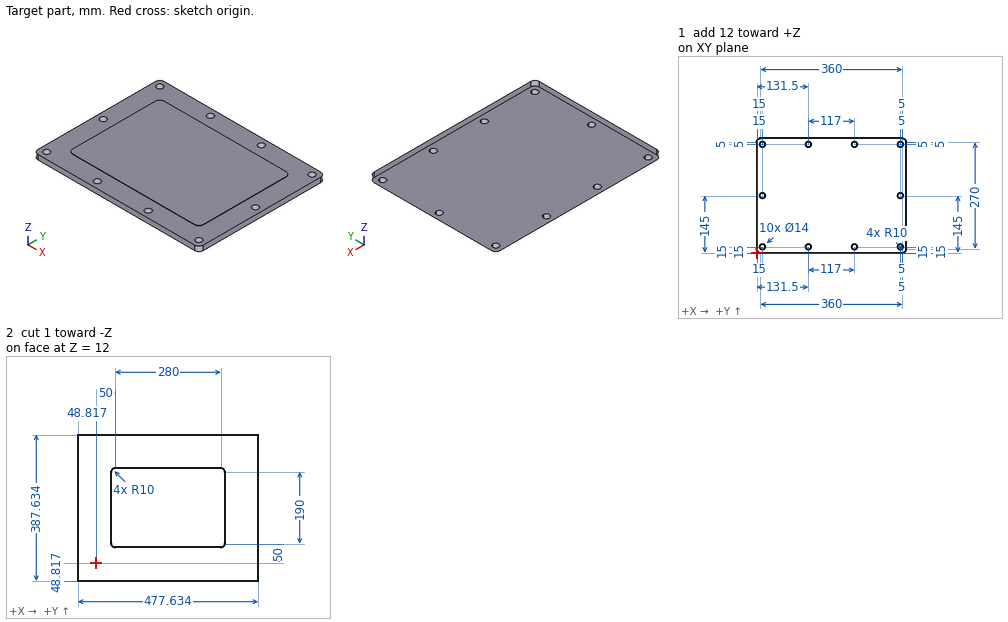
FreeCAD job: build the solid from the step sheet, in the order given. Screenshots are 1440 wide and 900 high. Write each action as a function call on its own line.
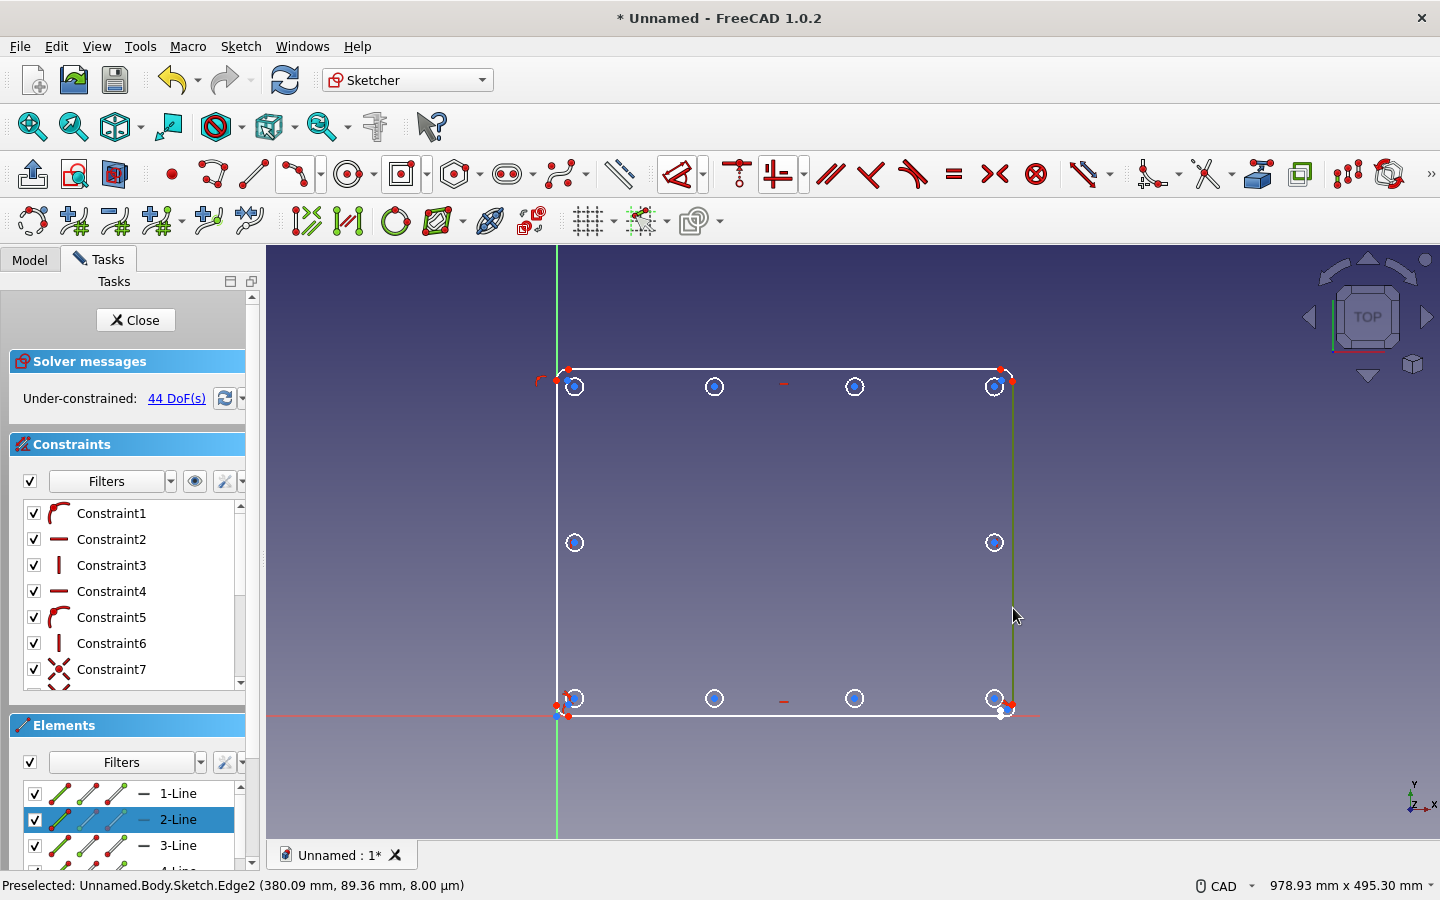
scroll(1010, 716, up, 4)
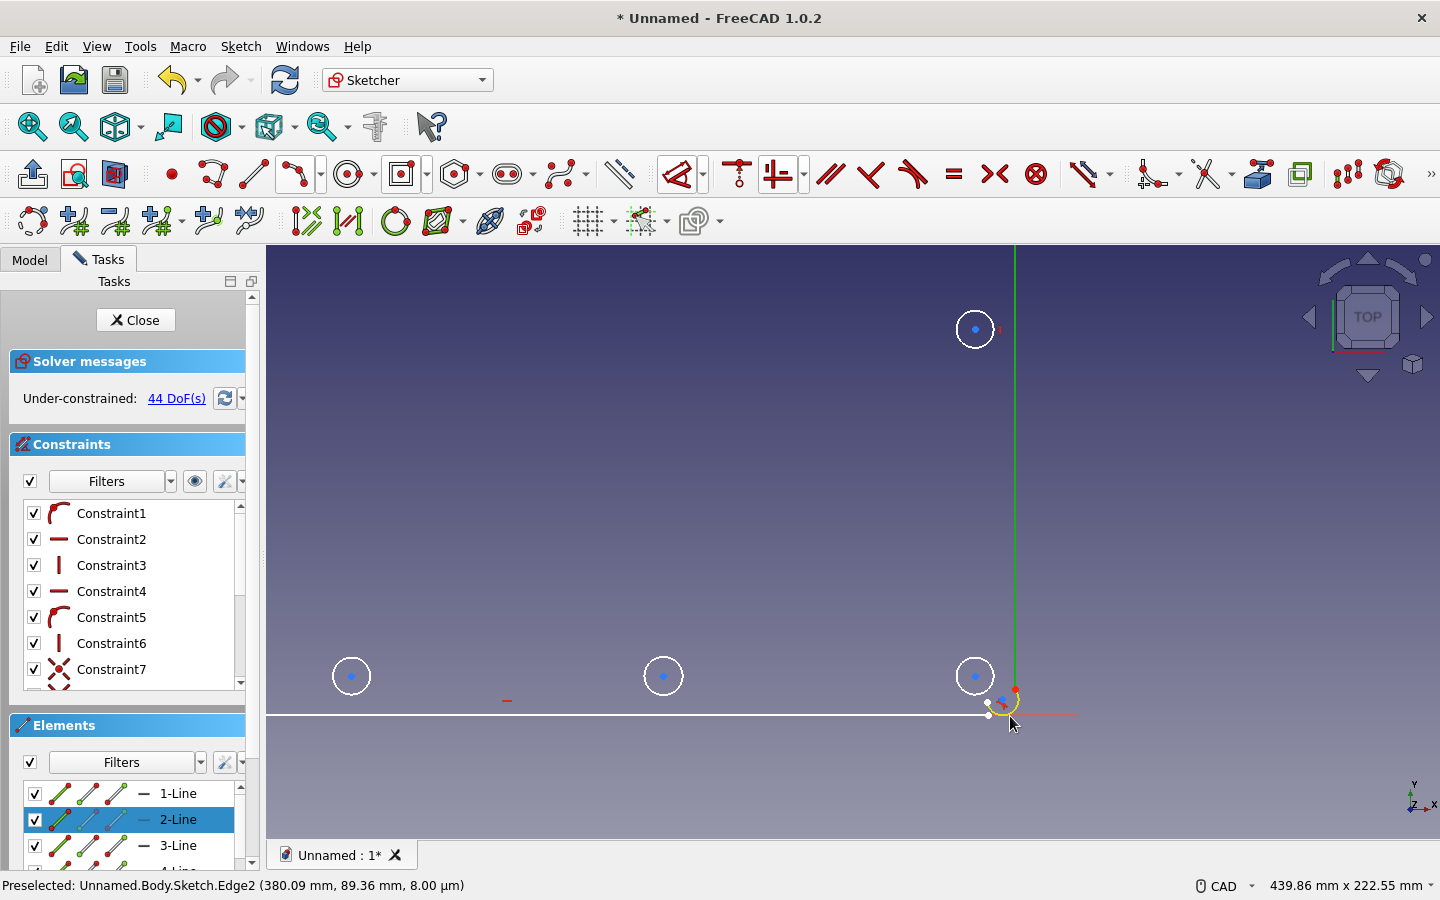
click(1009, 714)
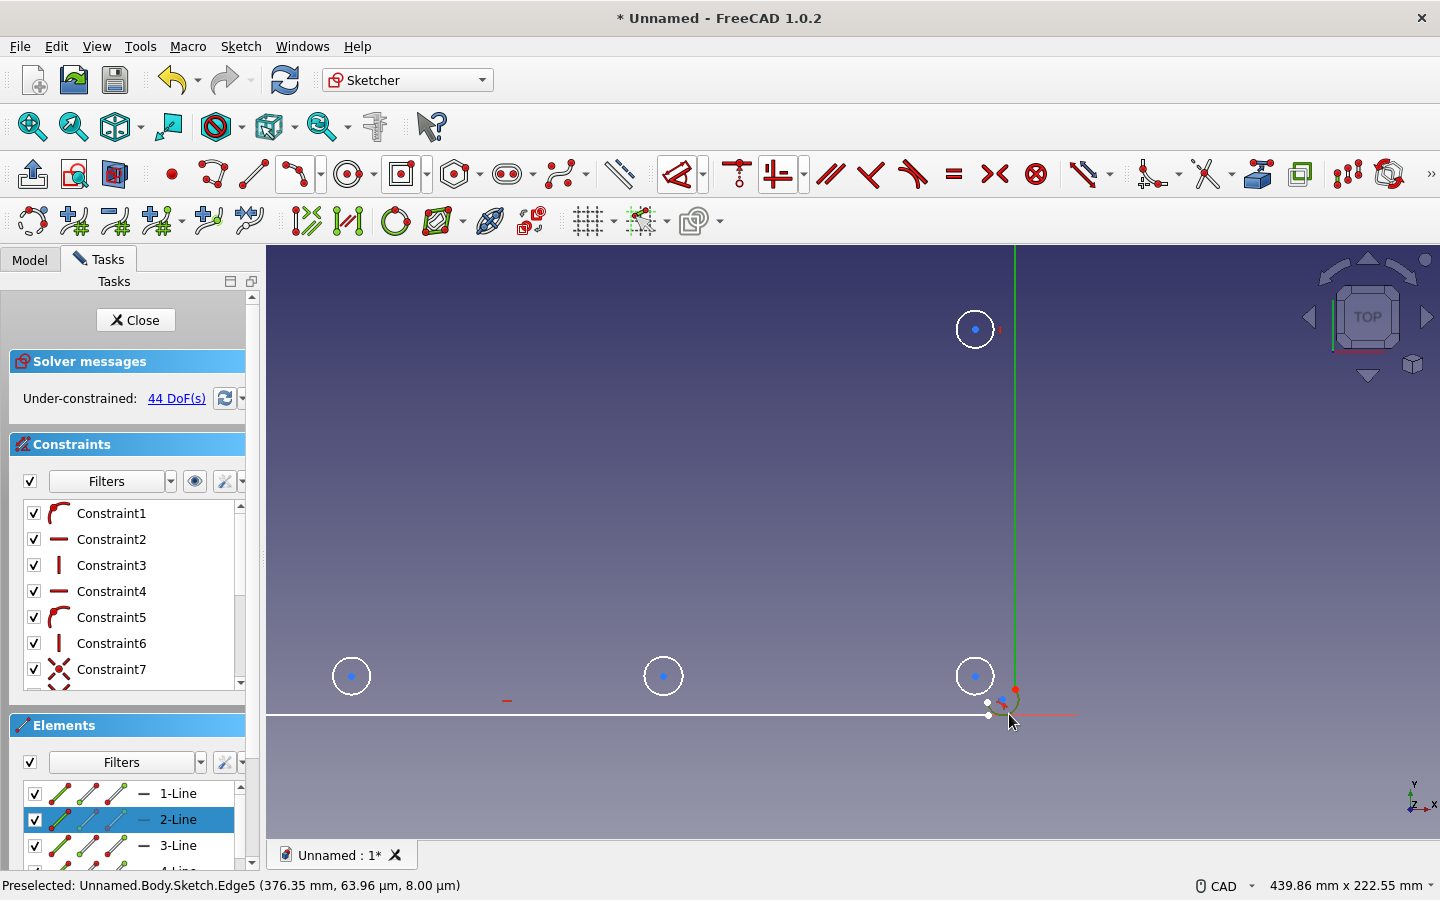
click(913, 174)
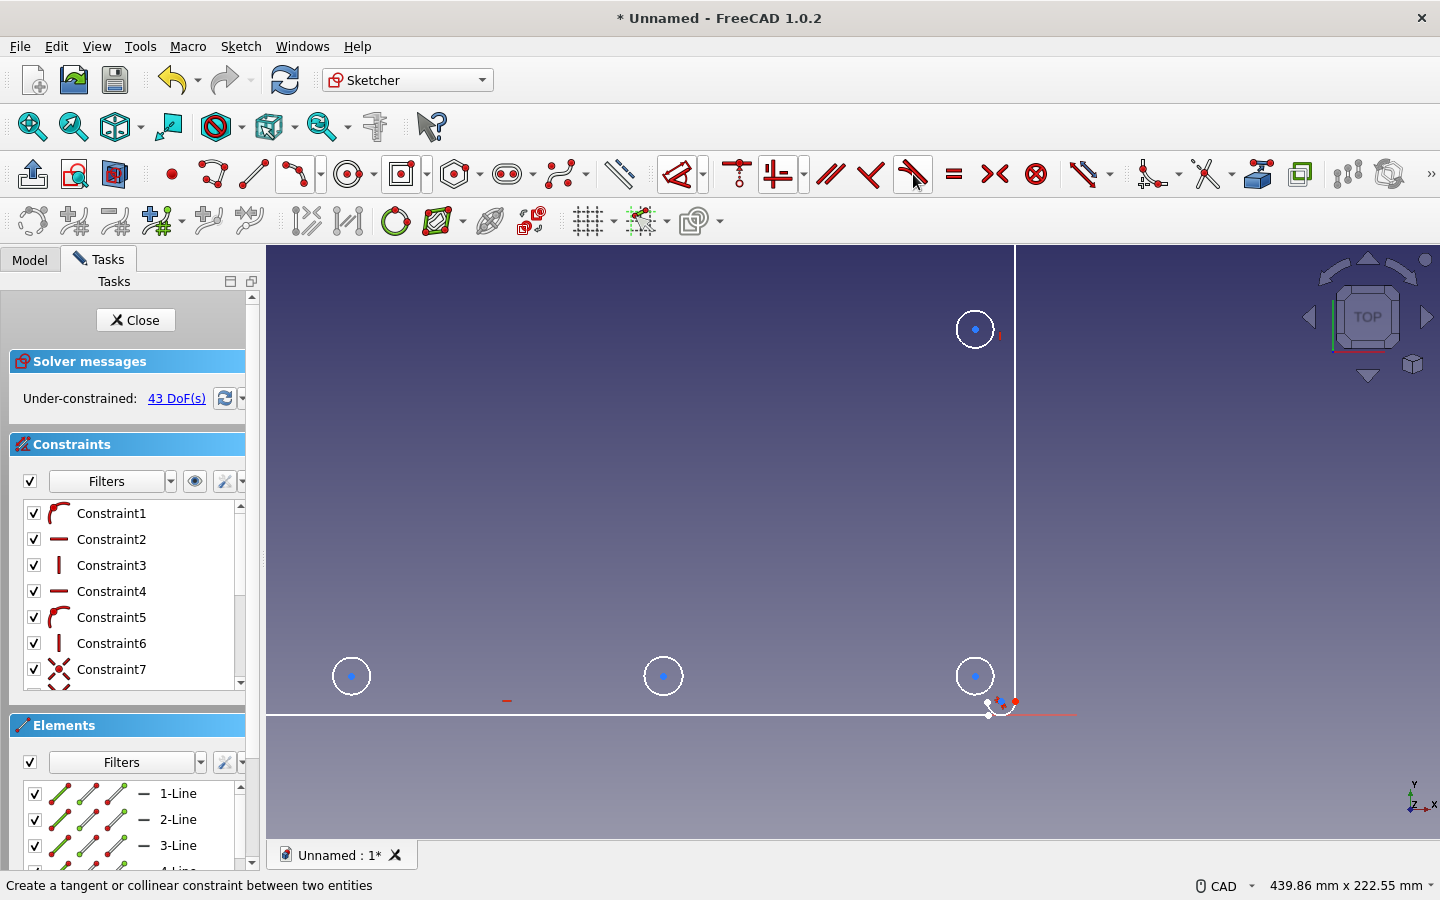
click(1015, 482)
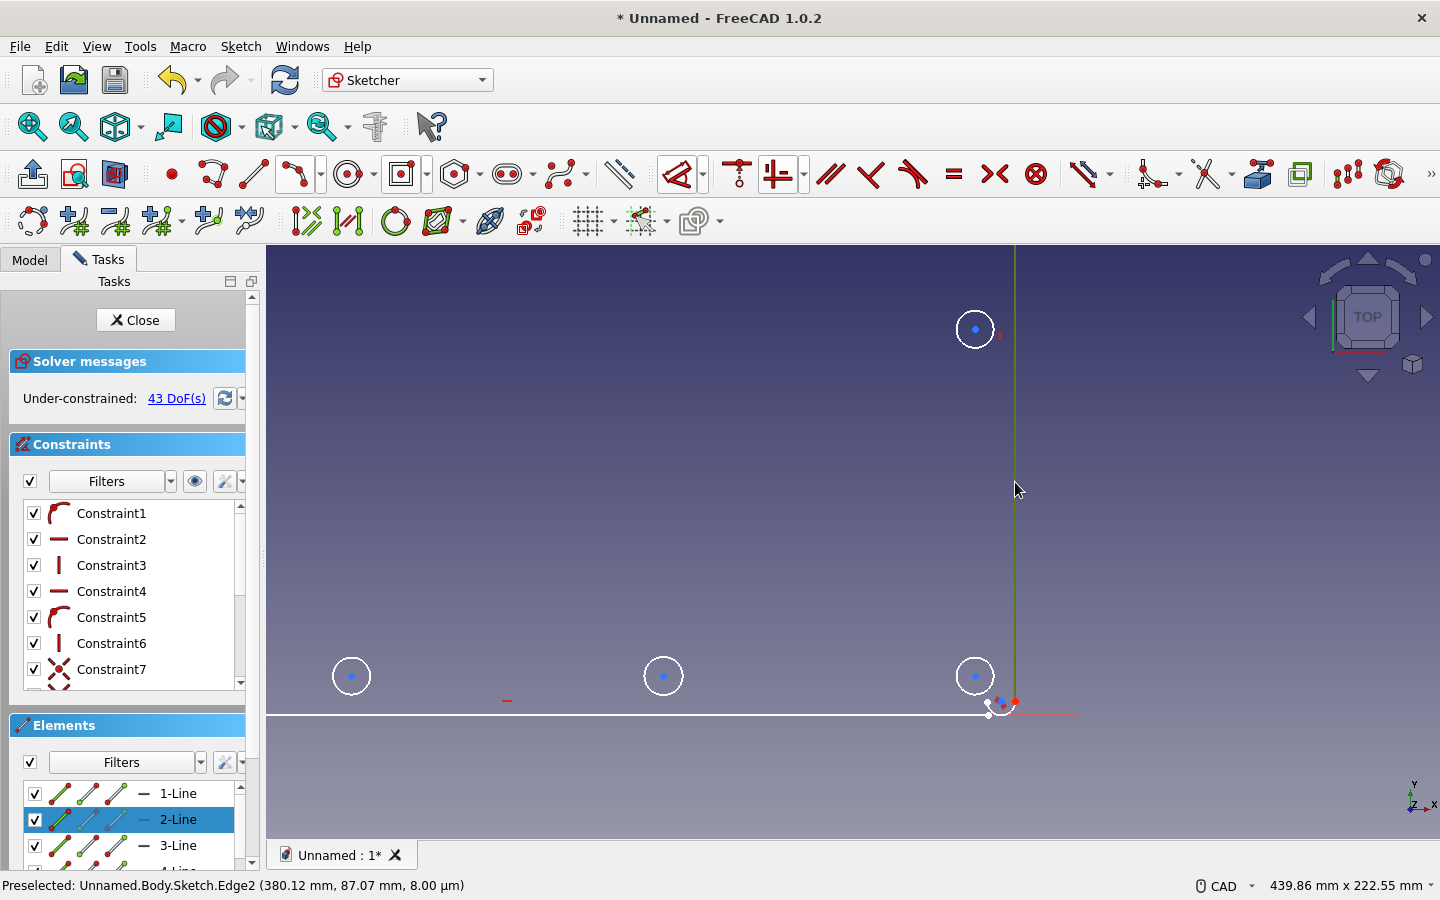
scroll(1010, 716, down, 4)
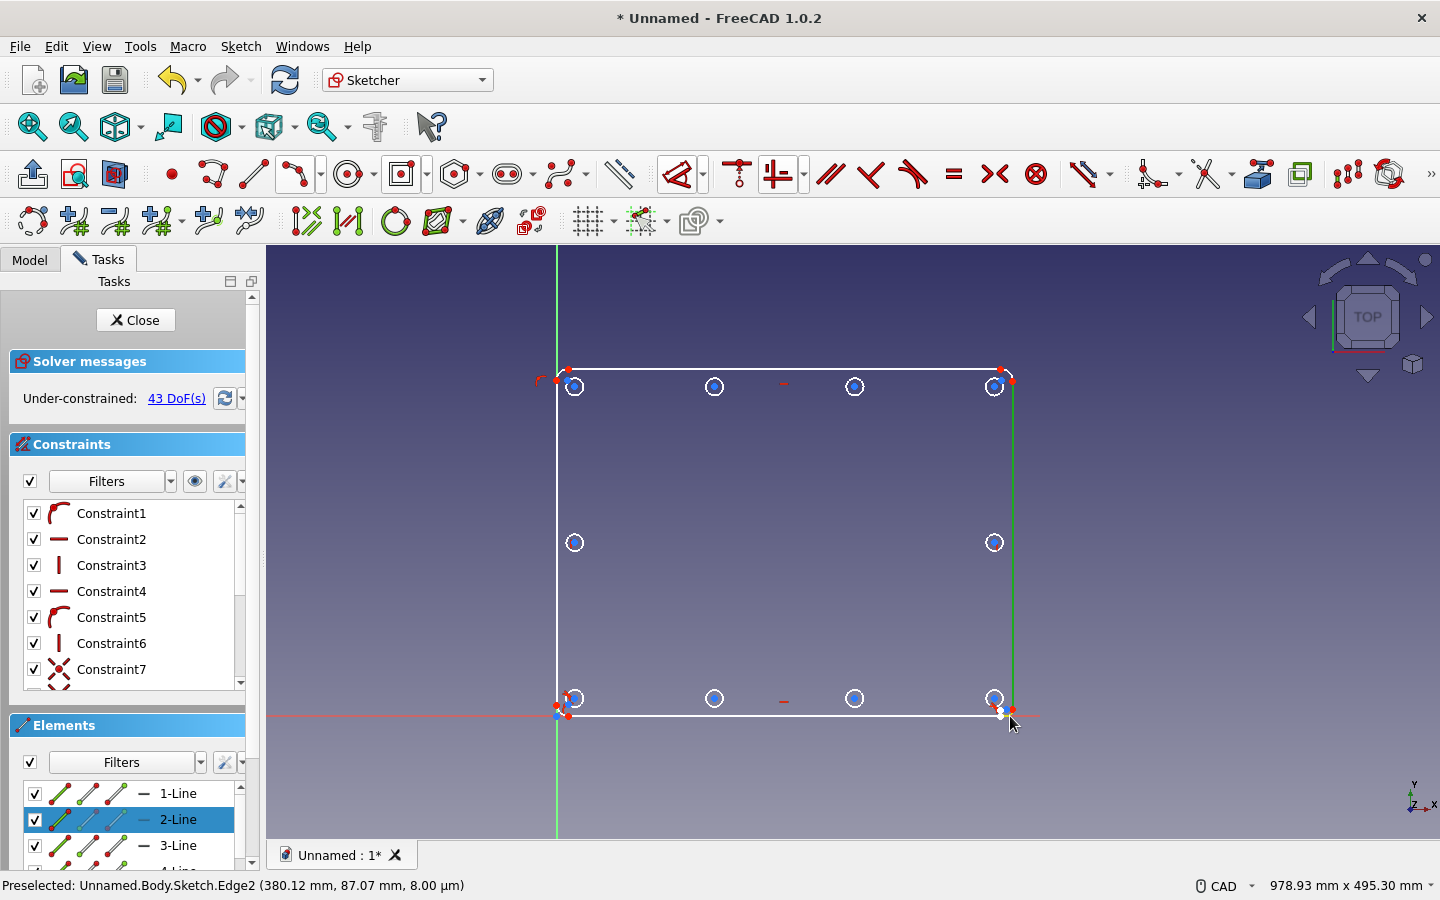
scroll(1012, 375, up, 5)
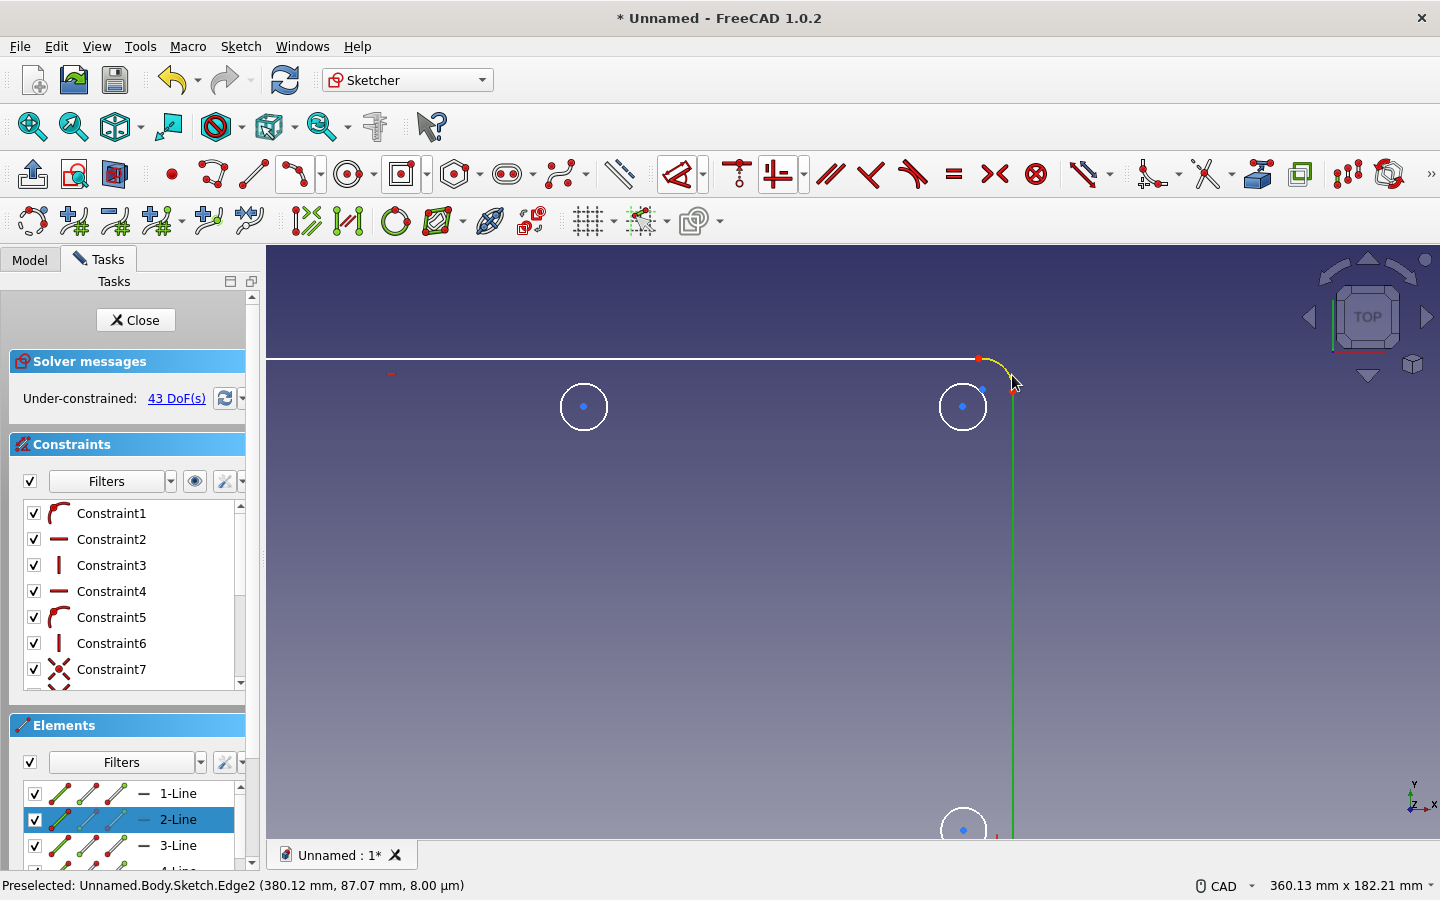
click(1010, 376)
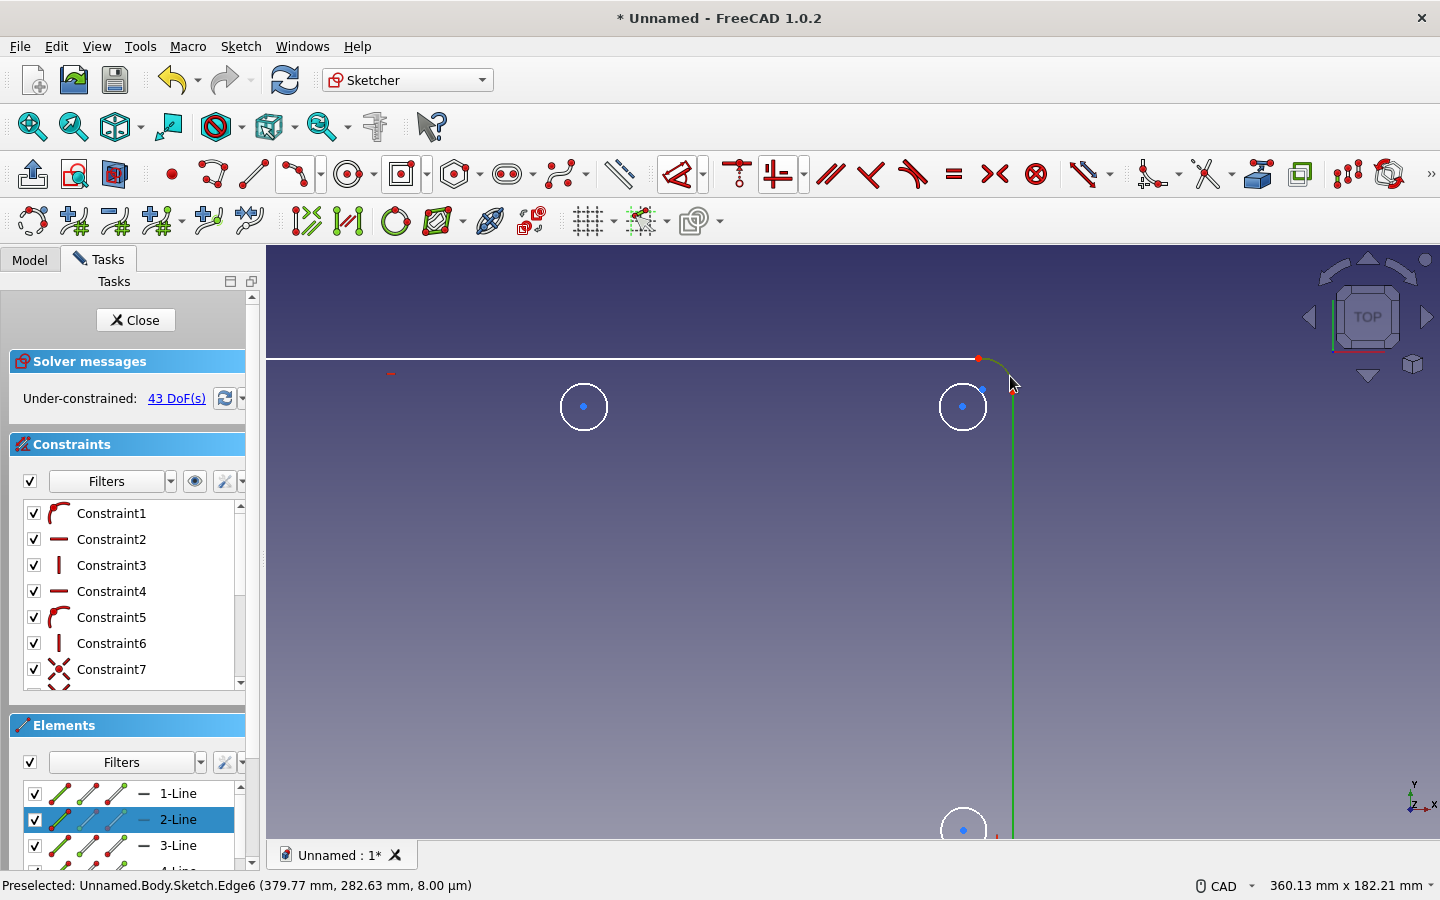
click(913, 174)